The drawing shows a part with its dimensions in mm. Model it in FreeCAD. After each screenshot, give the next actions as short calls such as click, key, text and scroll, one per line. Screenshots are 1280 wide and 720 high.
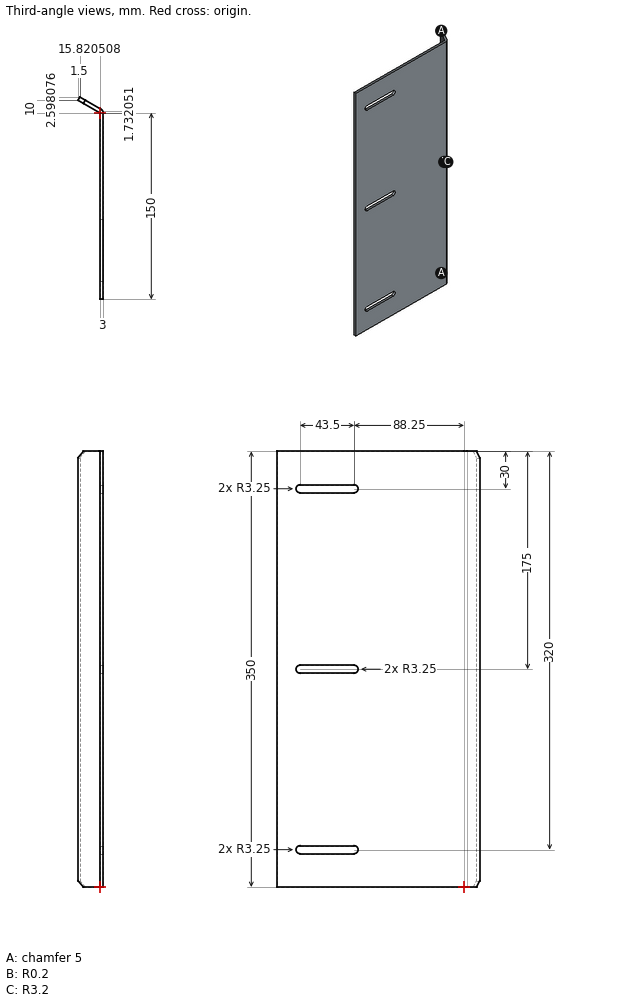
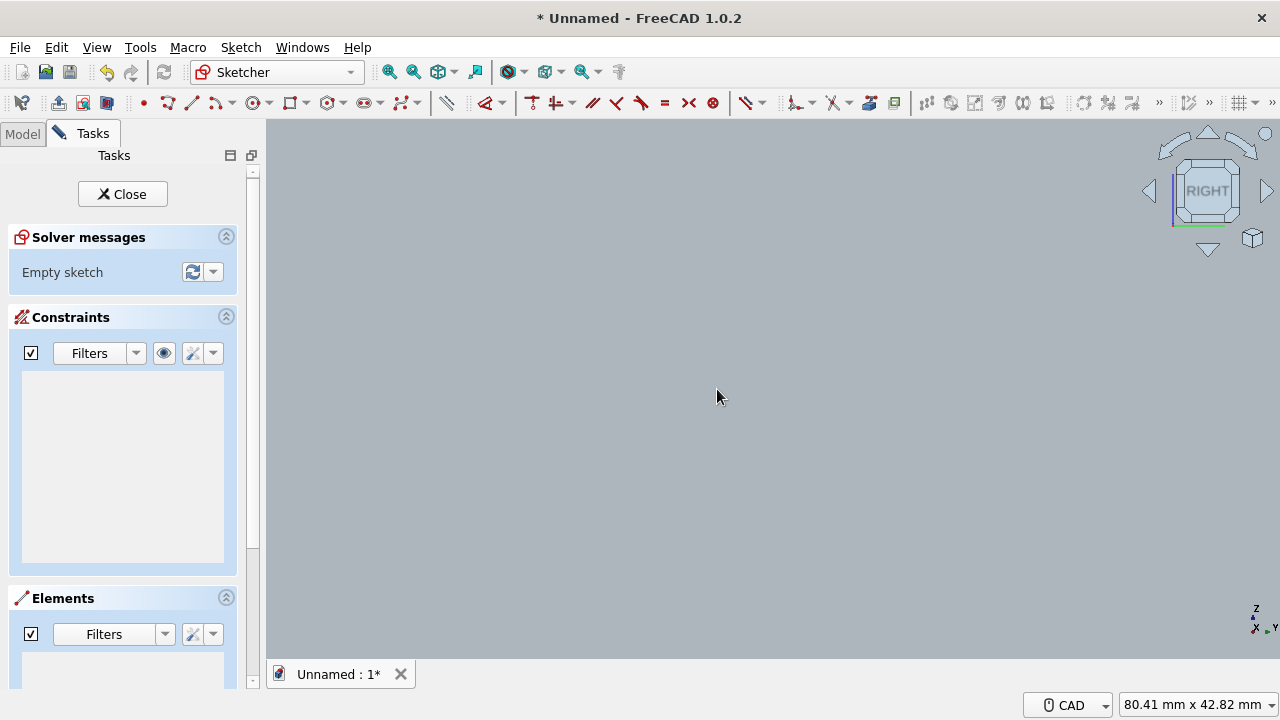
click(364, 104)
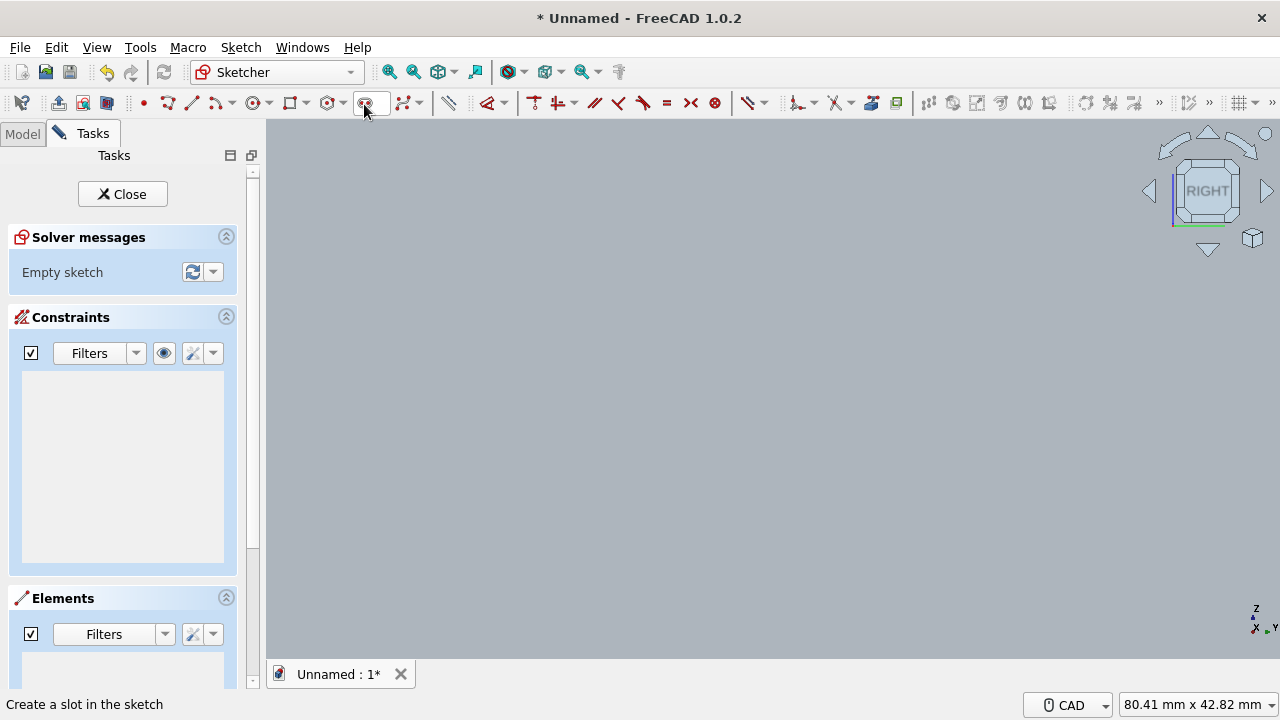
click(424, 385)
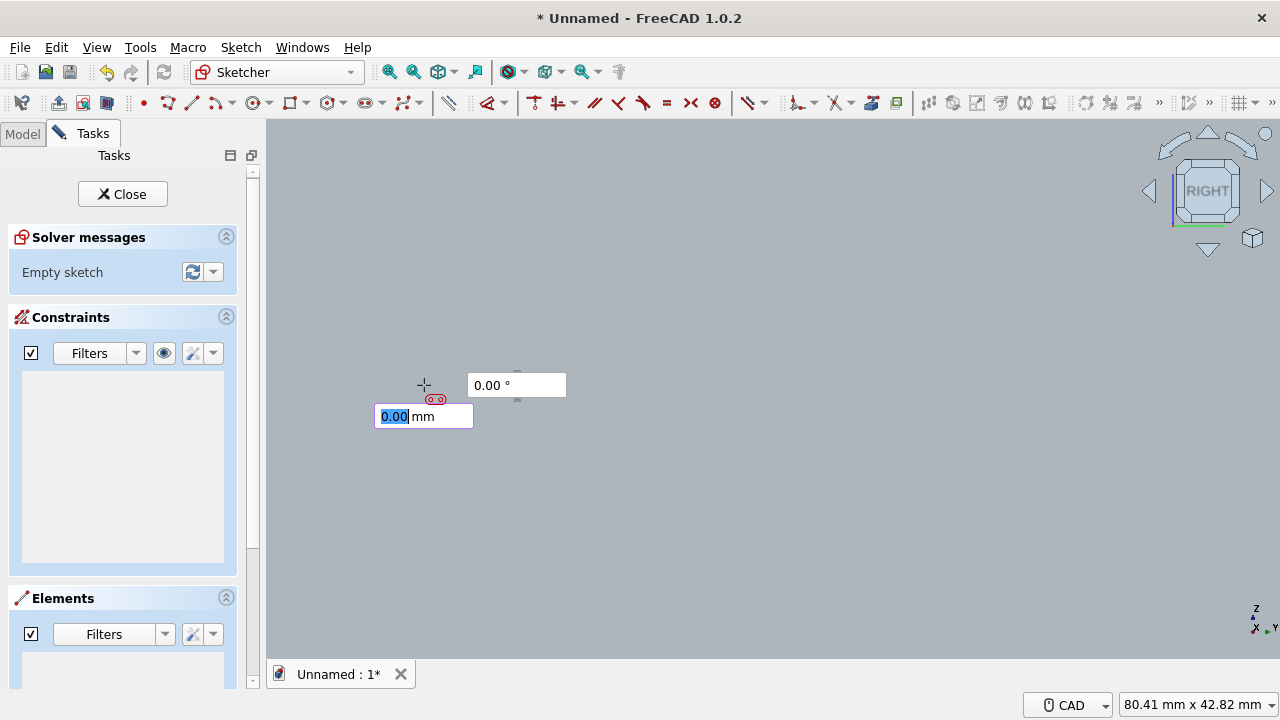
click(972, 385)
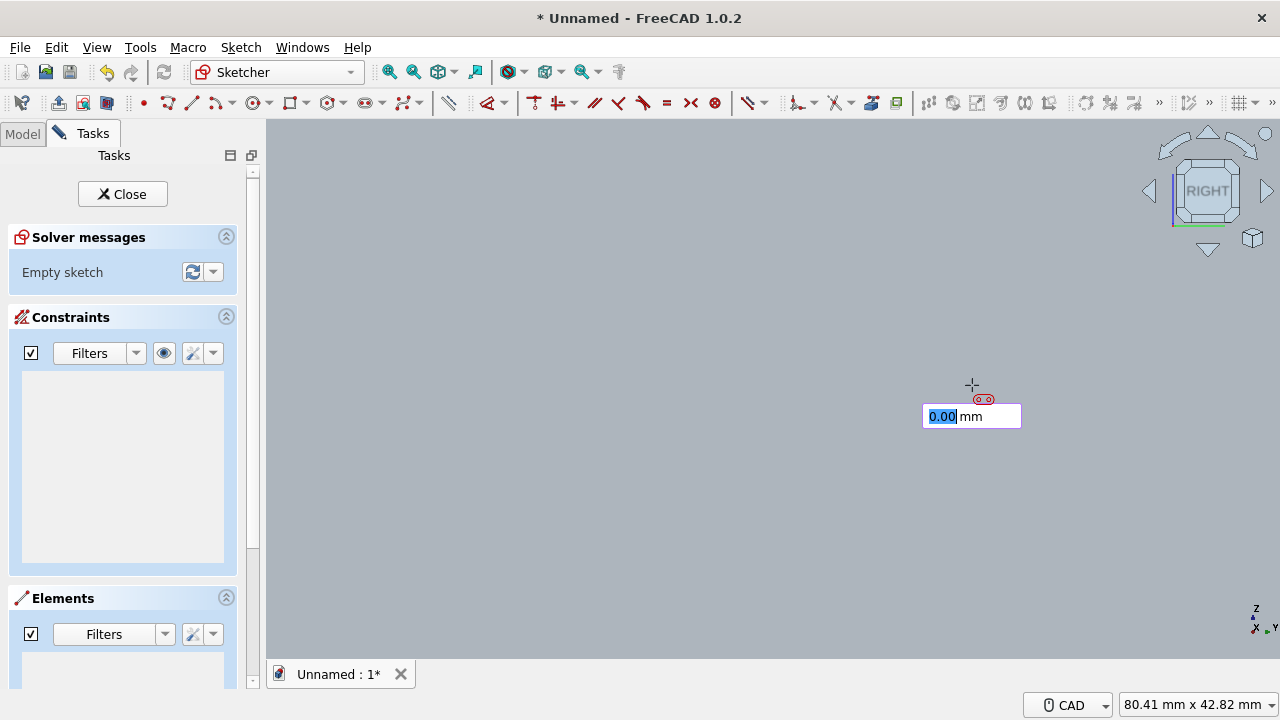
click(698, 426)
key(Escape)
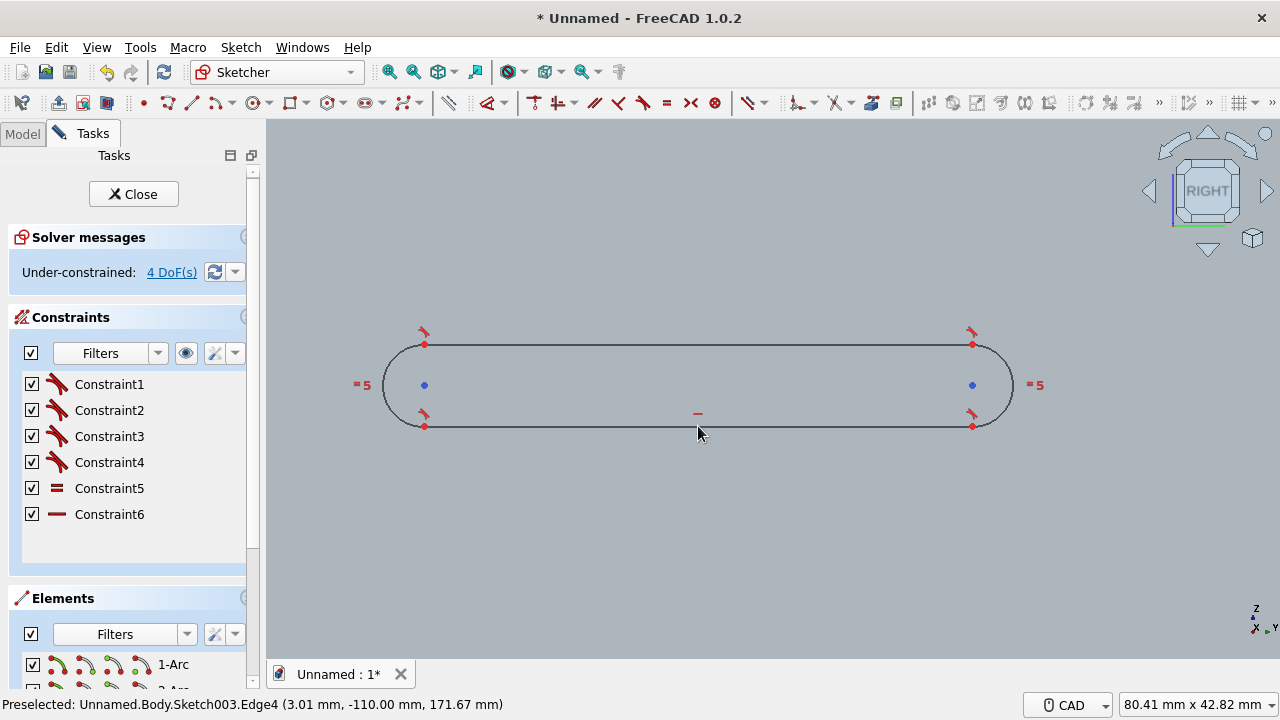
click(488, 104)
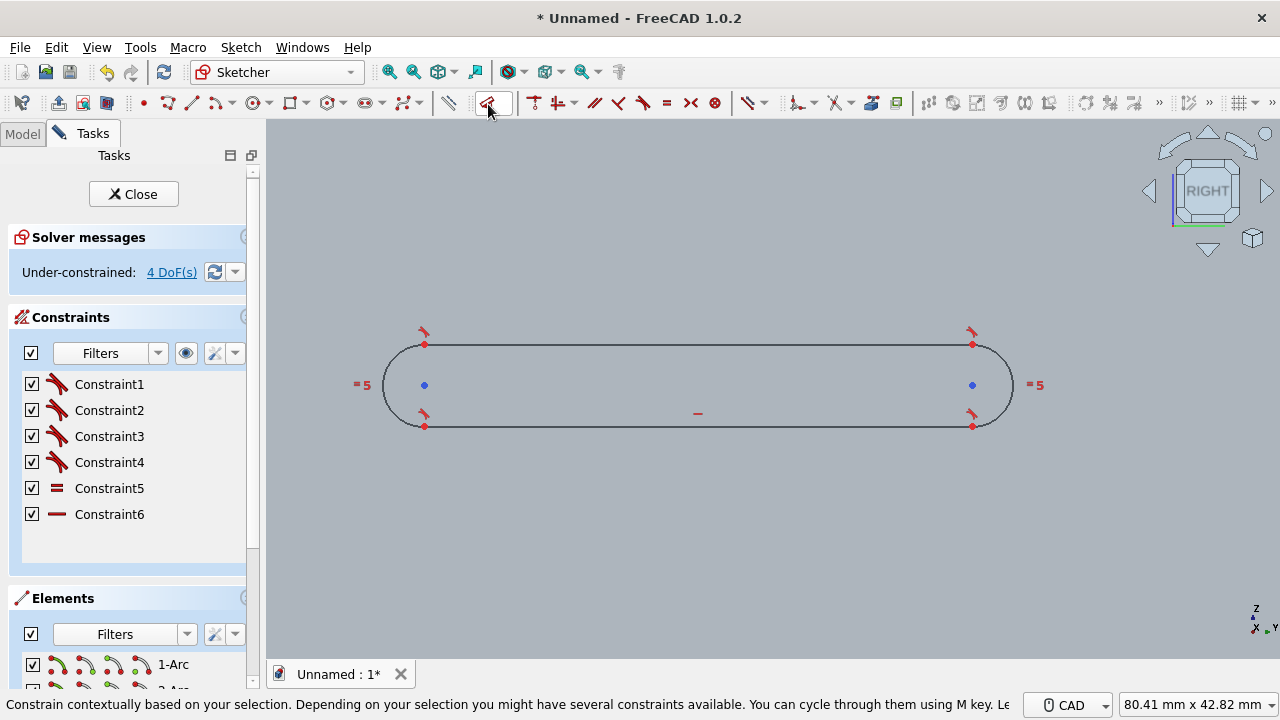
click(391, 362)
click(365, 343)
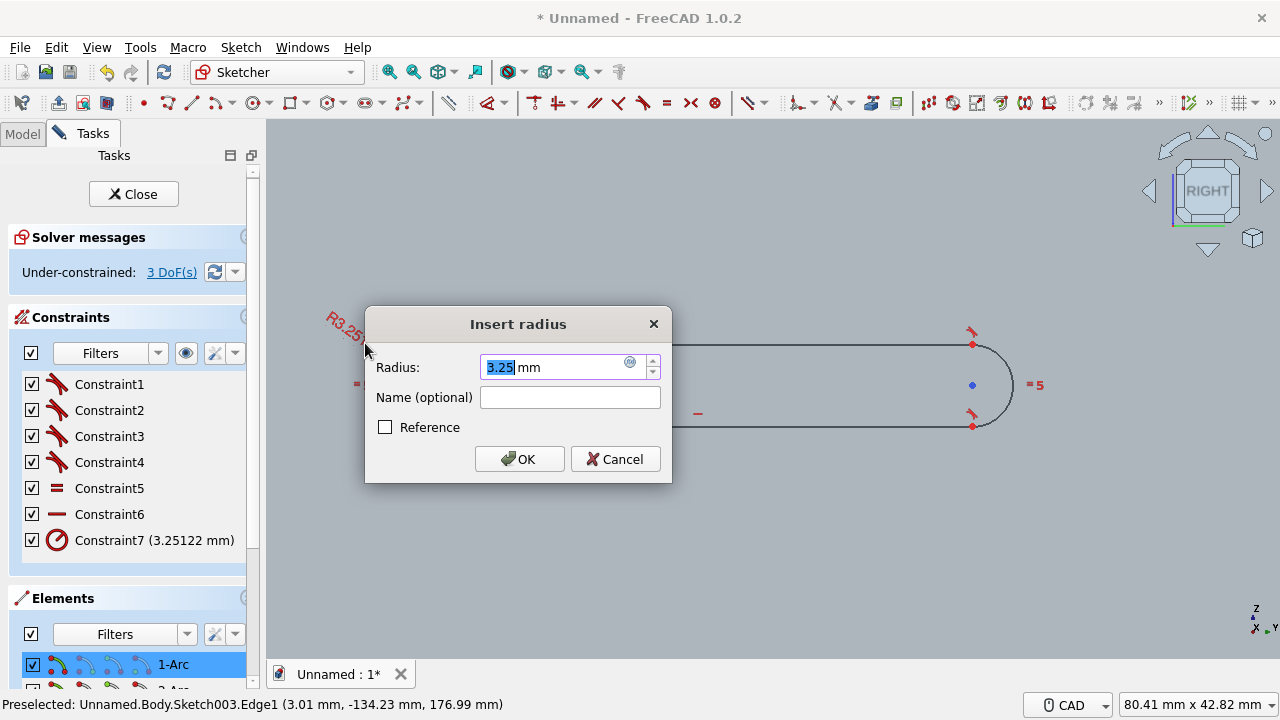
text(3.25)
key(Return)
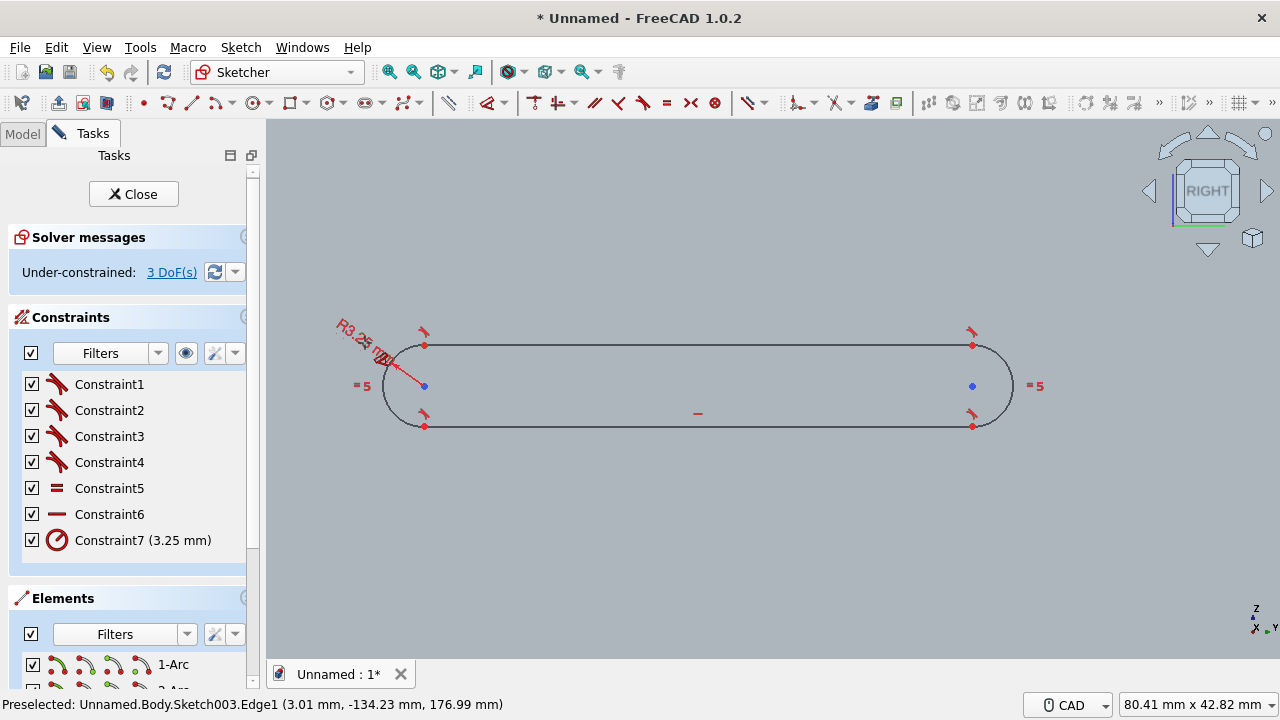
click(588, 345)
click(698, 311)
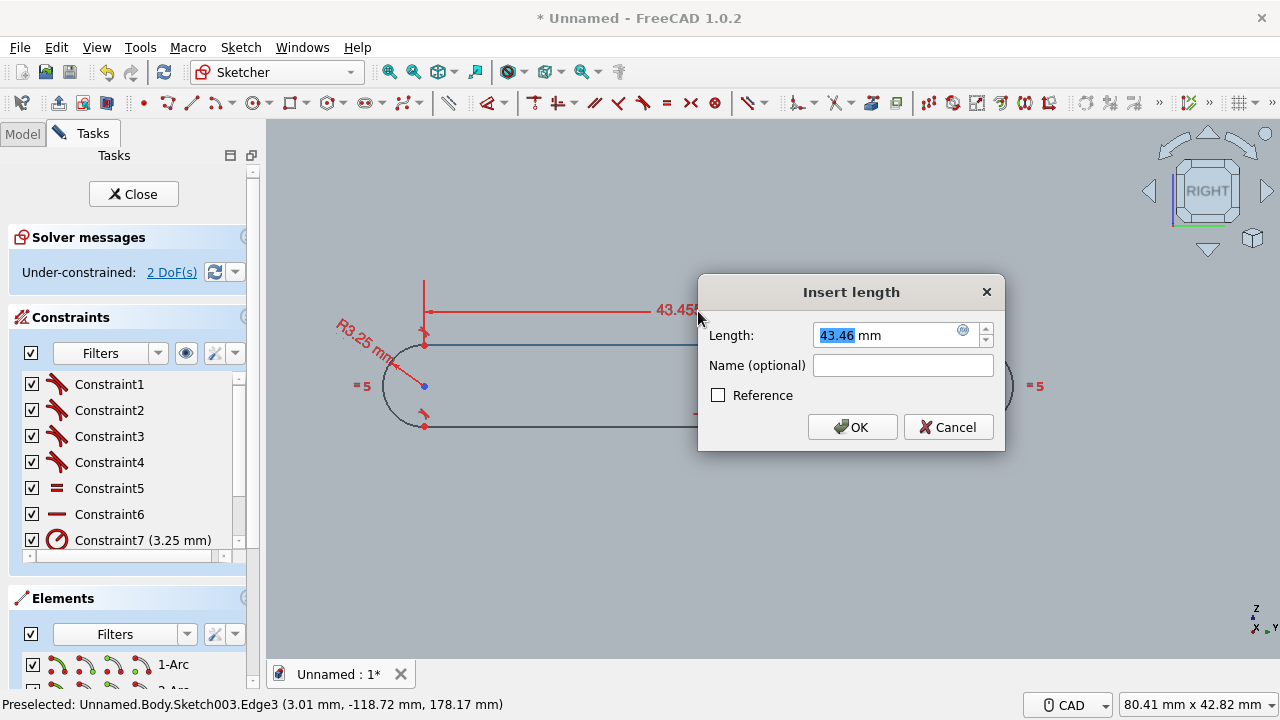
text(43.5)
key(Return)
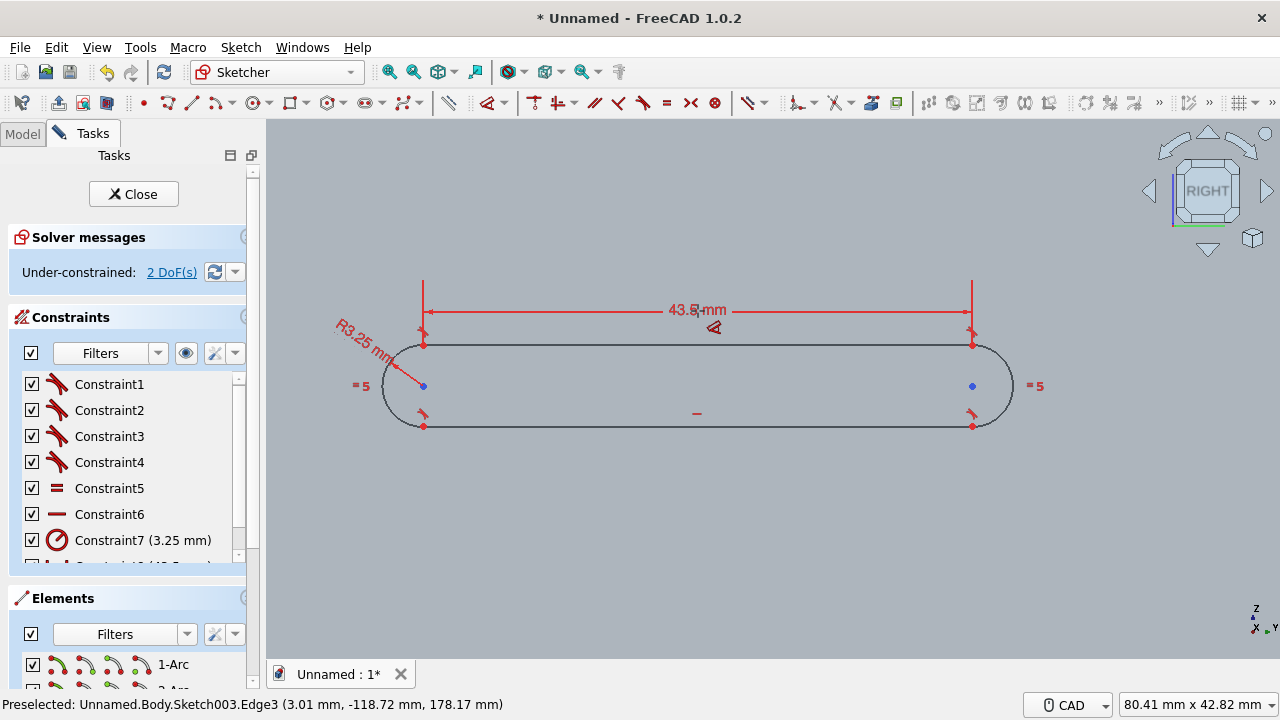
click(423, 386)
click(389, 267)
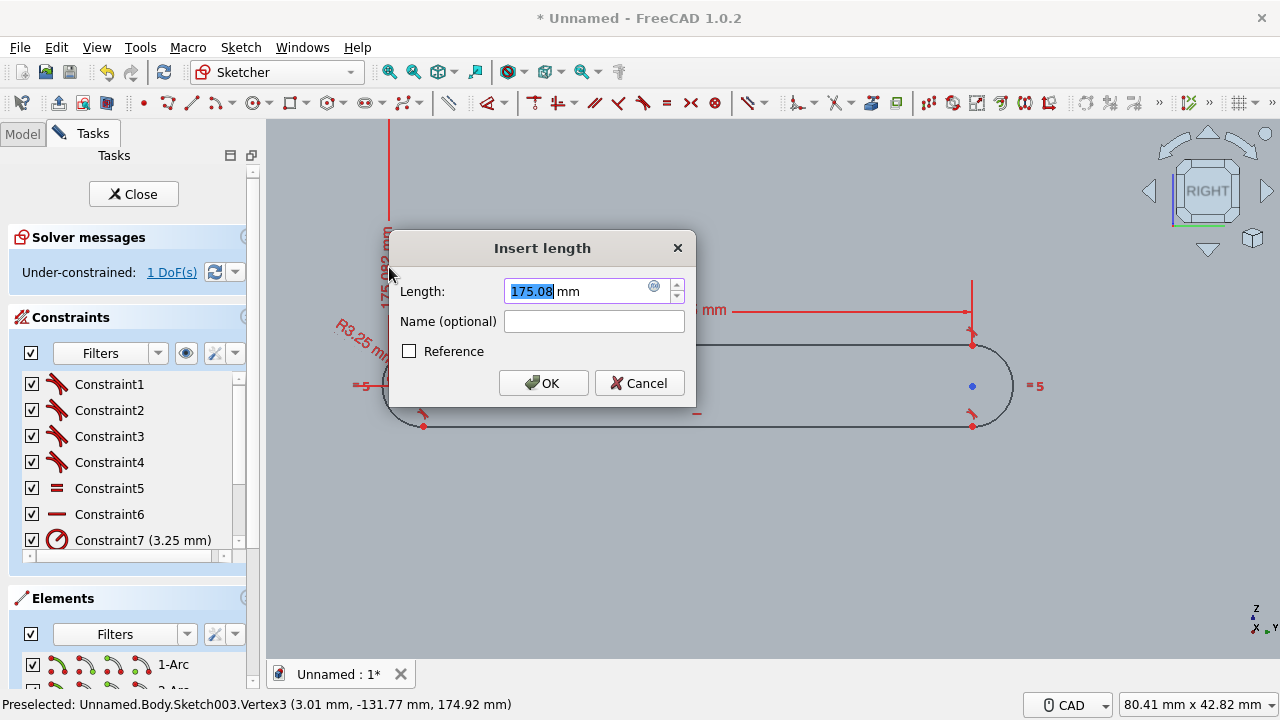
text(175)
key(Return)